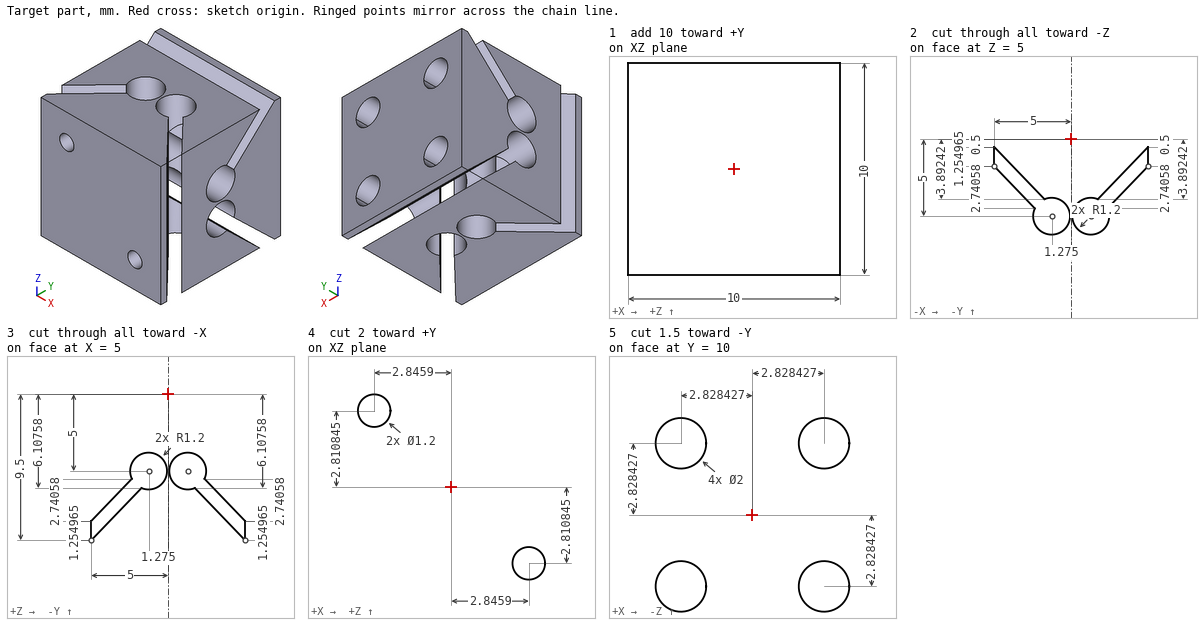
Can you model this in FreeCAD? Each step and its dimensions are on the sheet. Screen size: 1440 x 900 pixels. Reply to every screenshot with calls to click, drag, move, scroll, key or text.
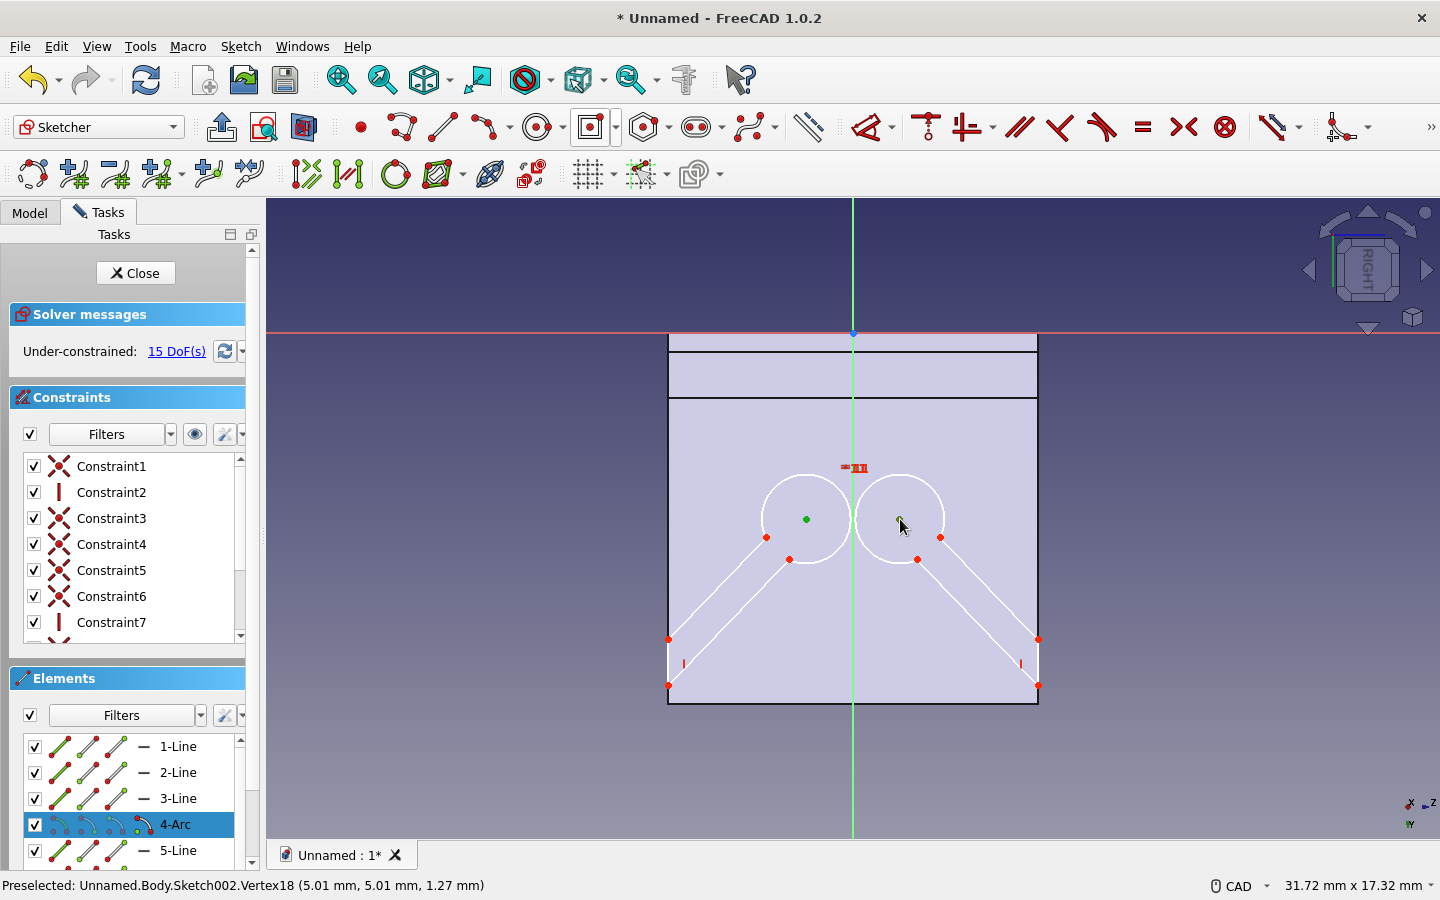
click(853, 769)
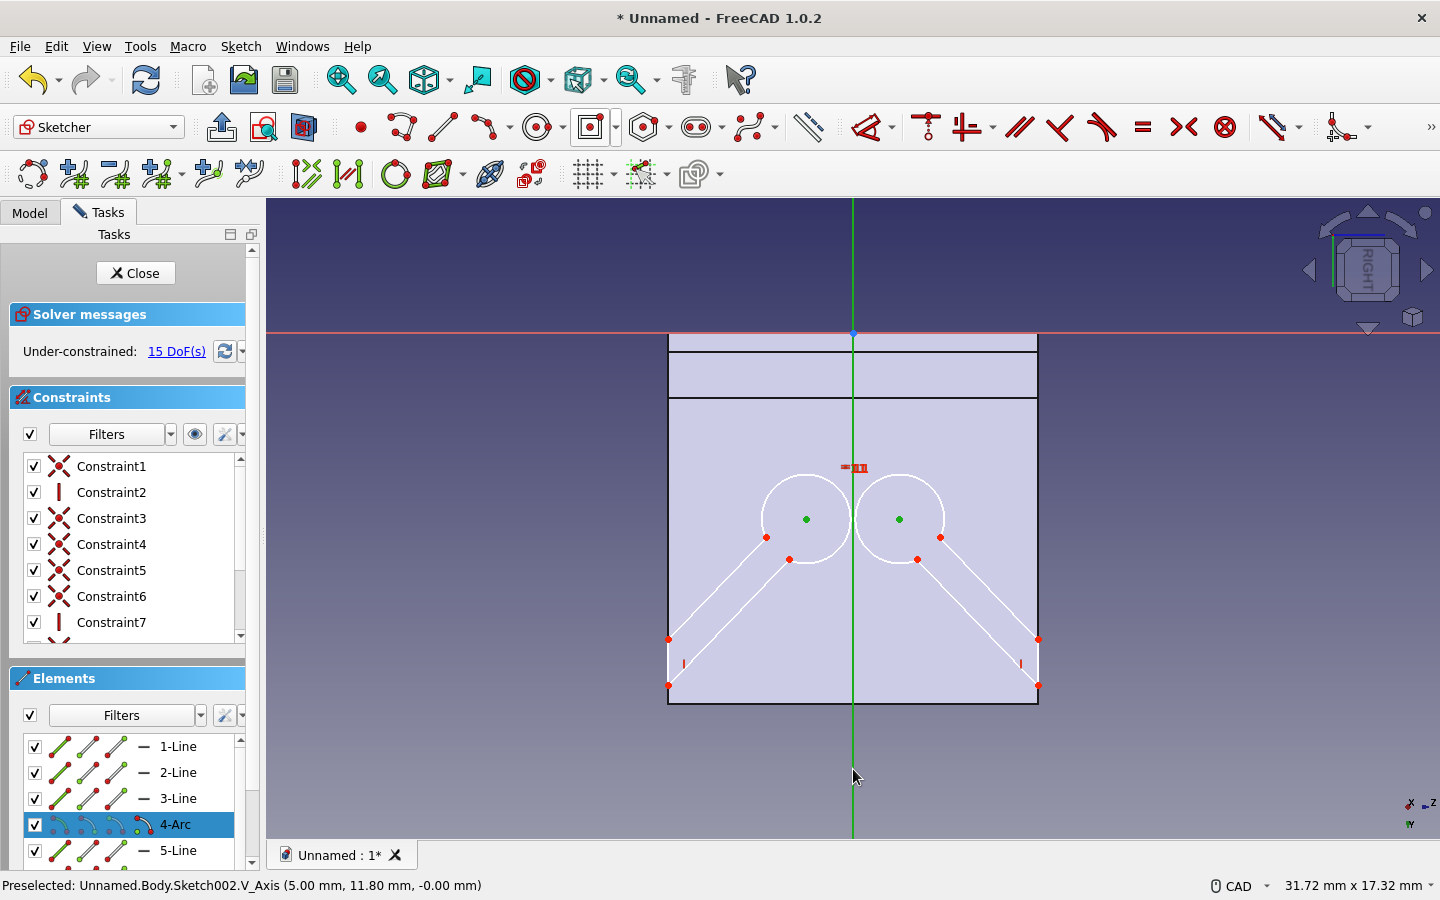
click(1184, 128)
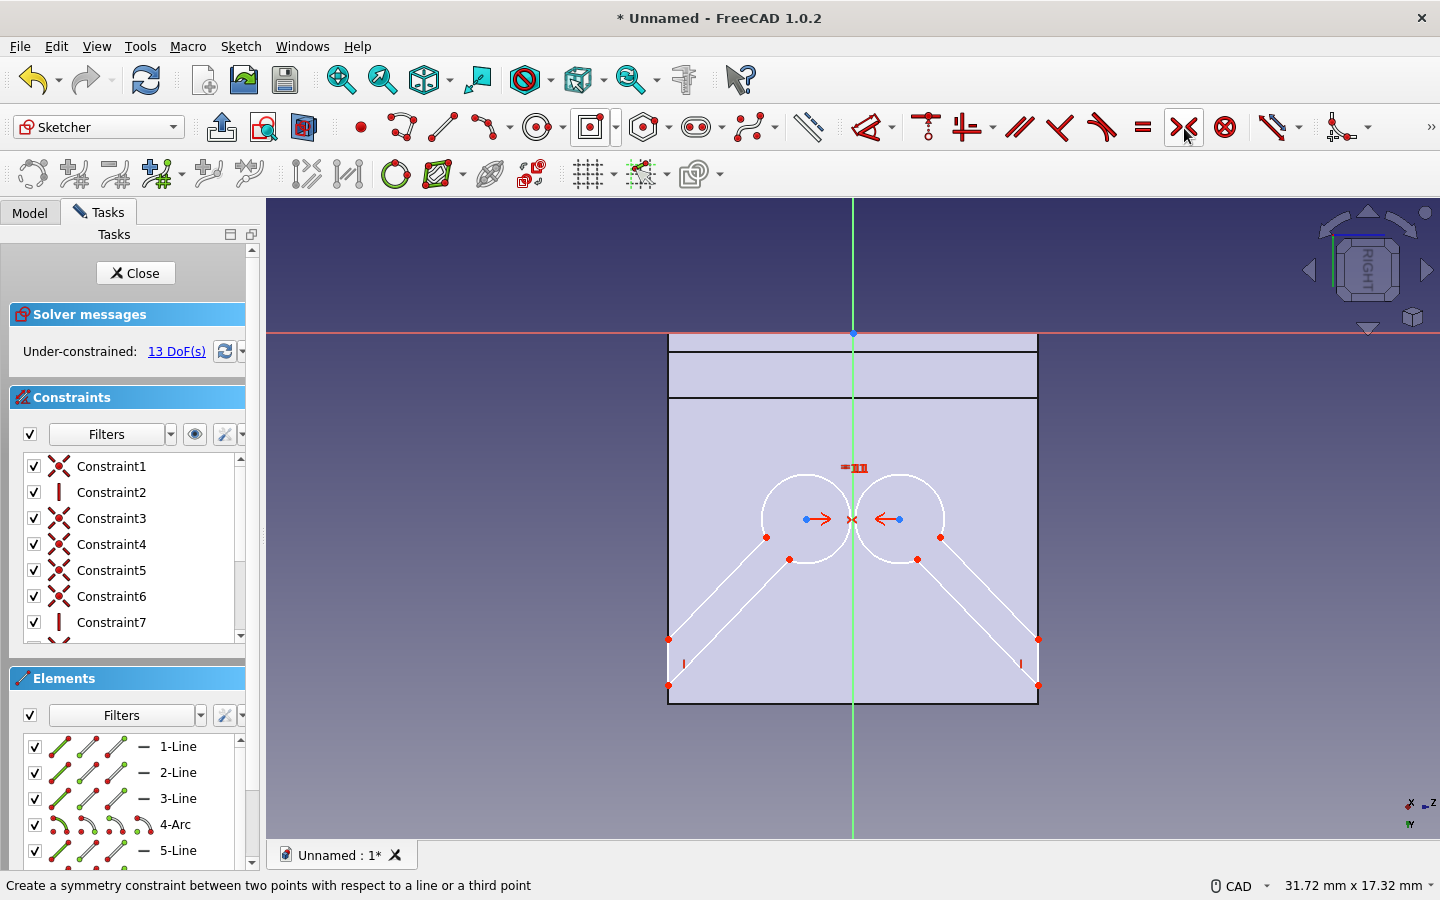
click(668, 686)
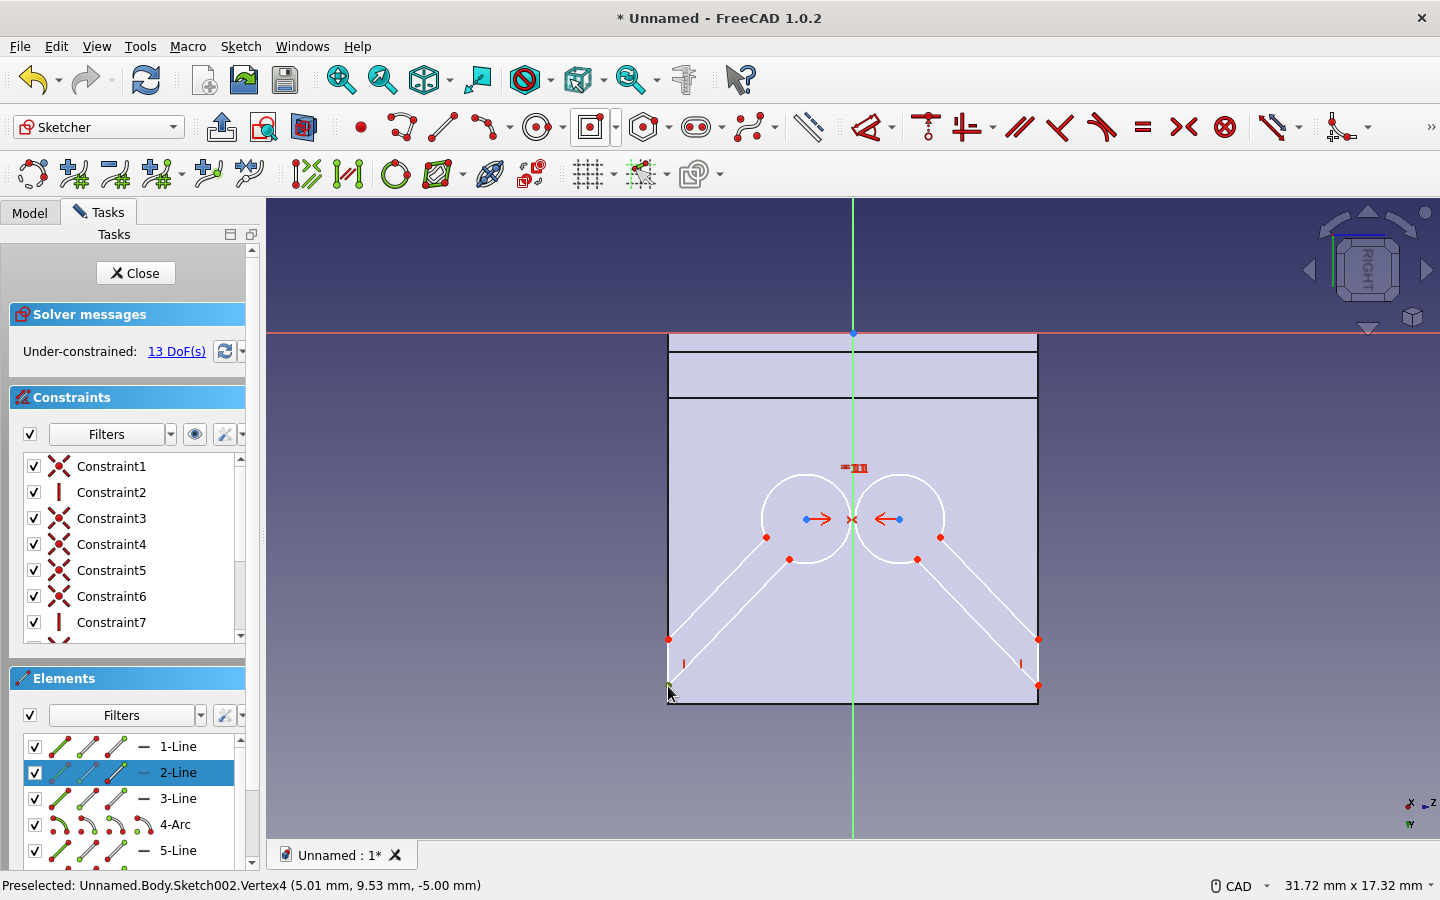
click(1038, 686)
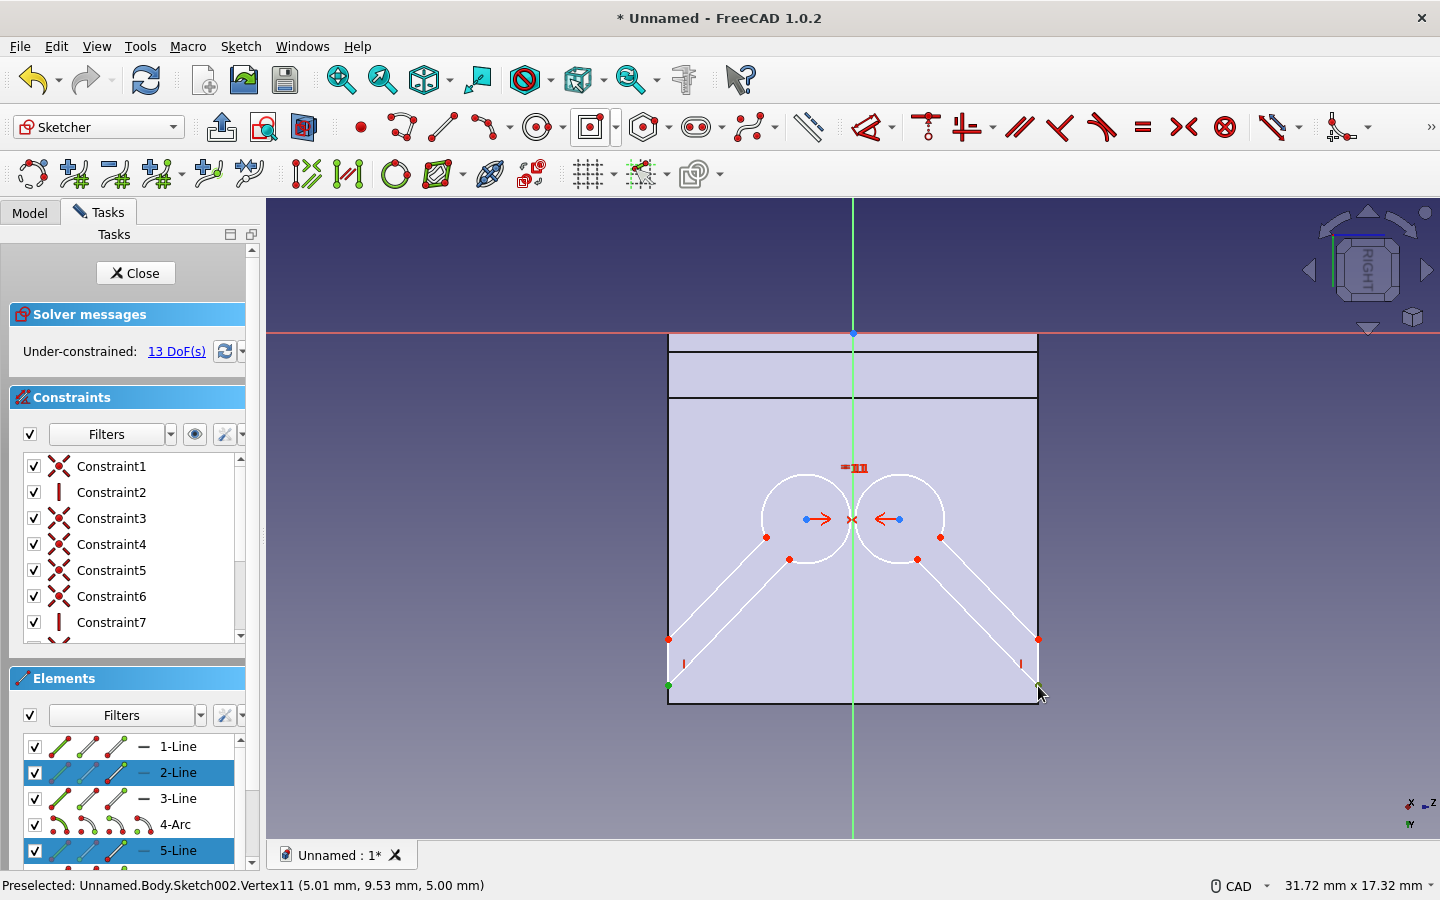
click(853, 769)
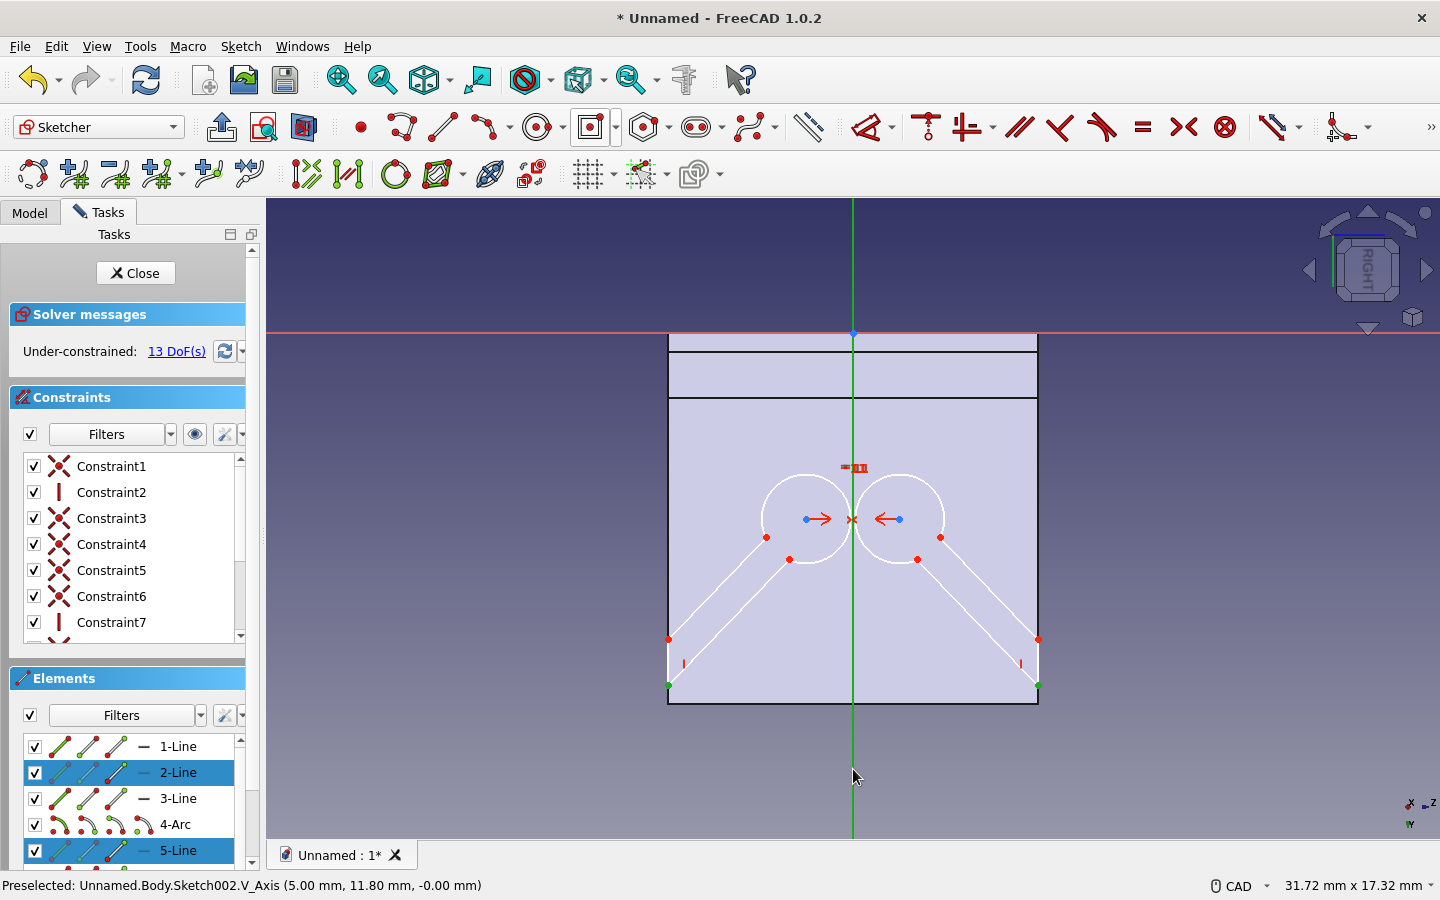
key(s)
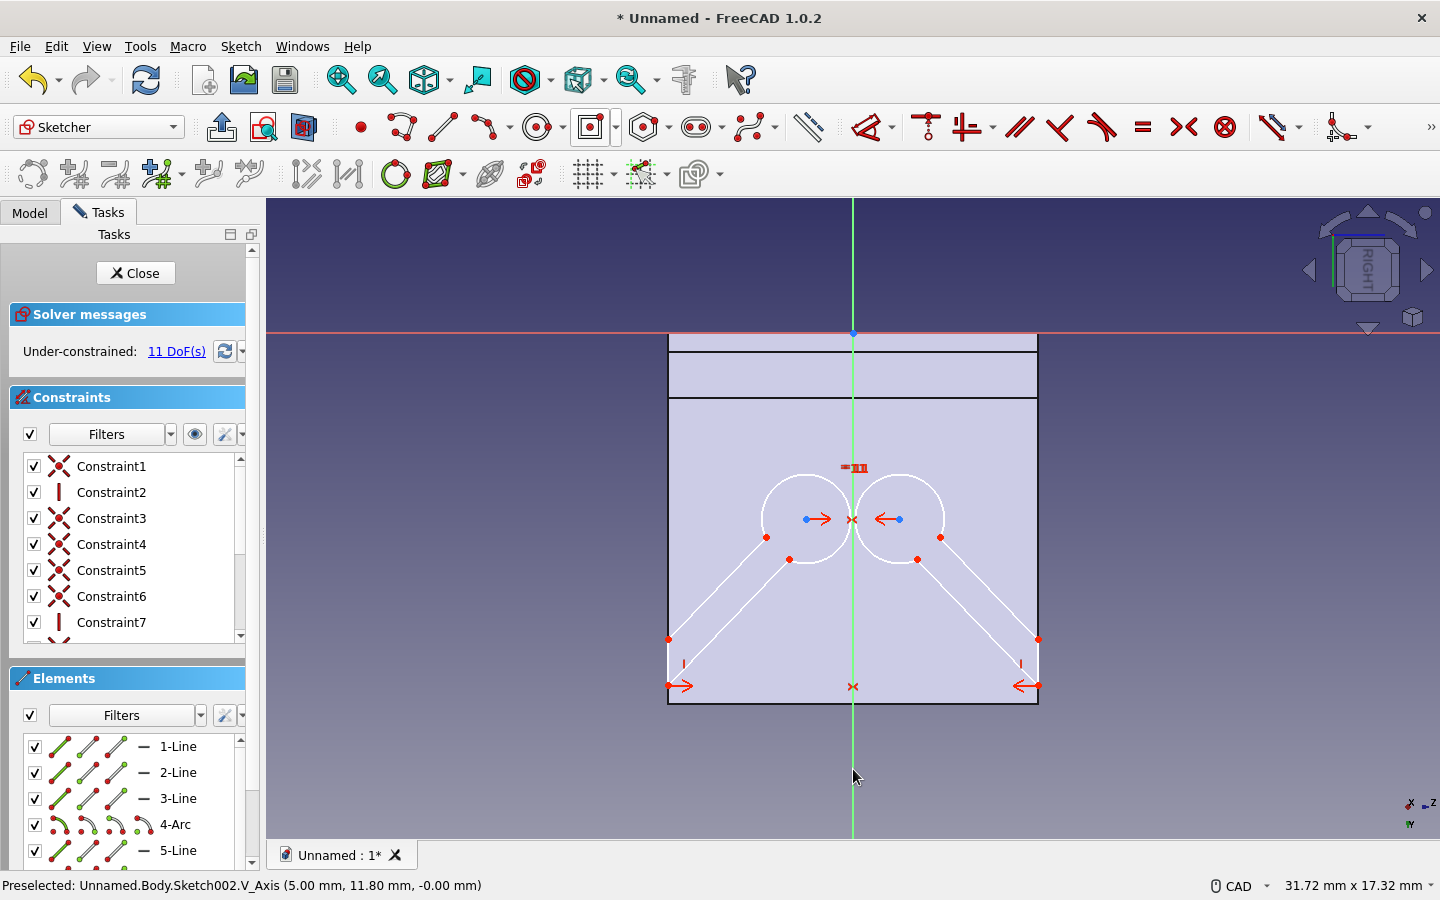
key(d)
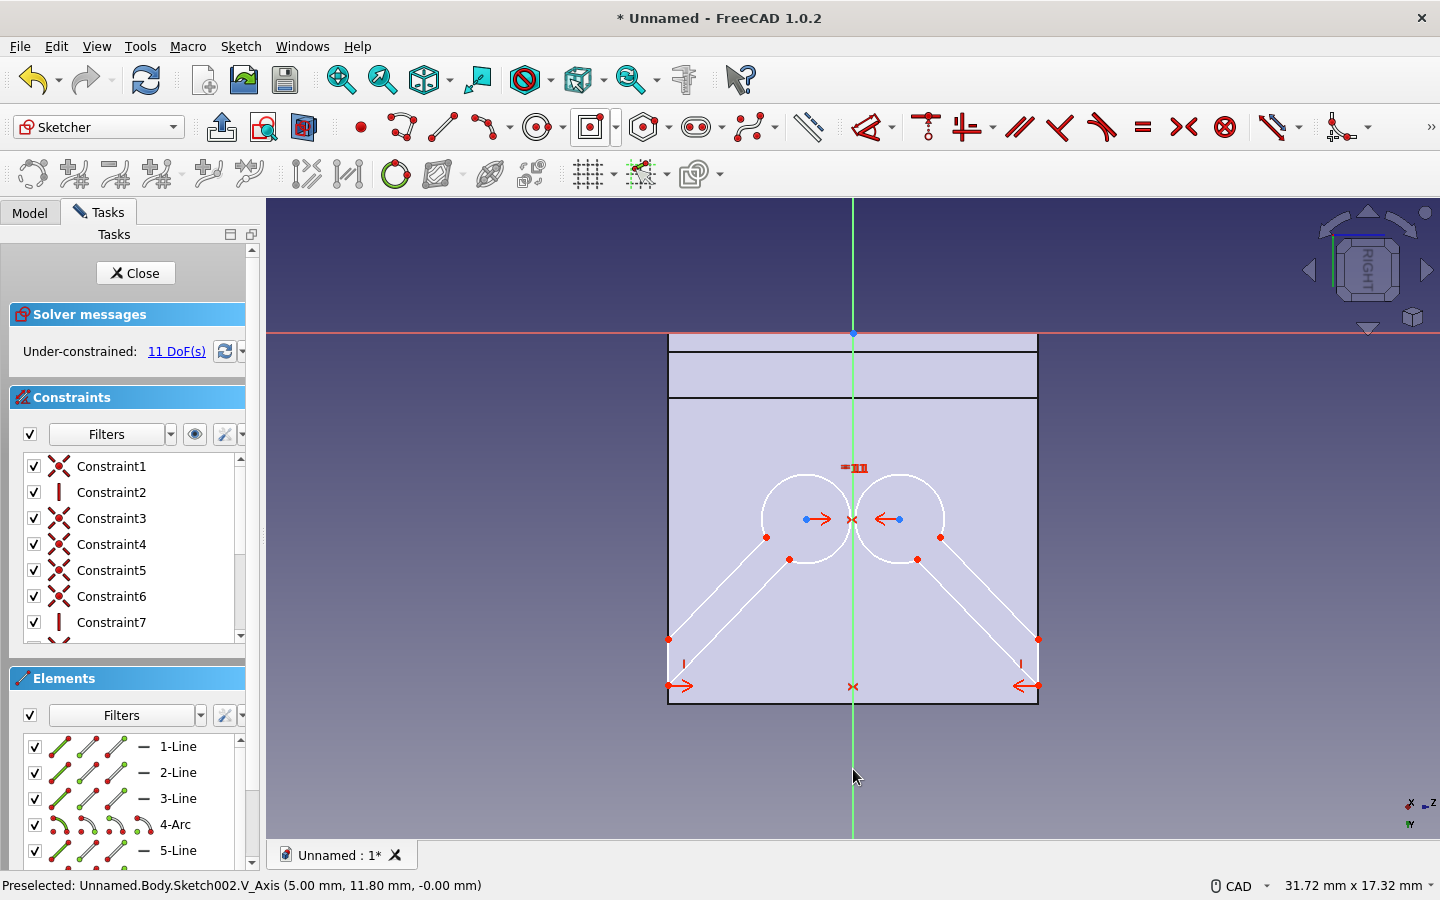
click(791, 477)
click(780, 447)